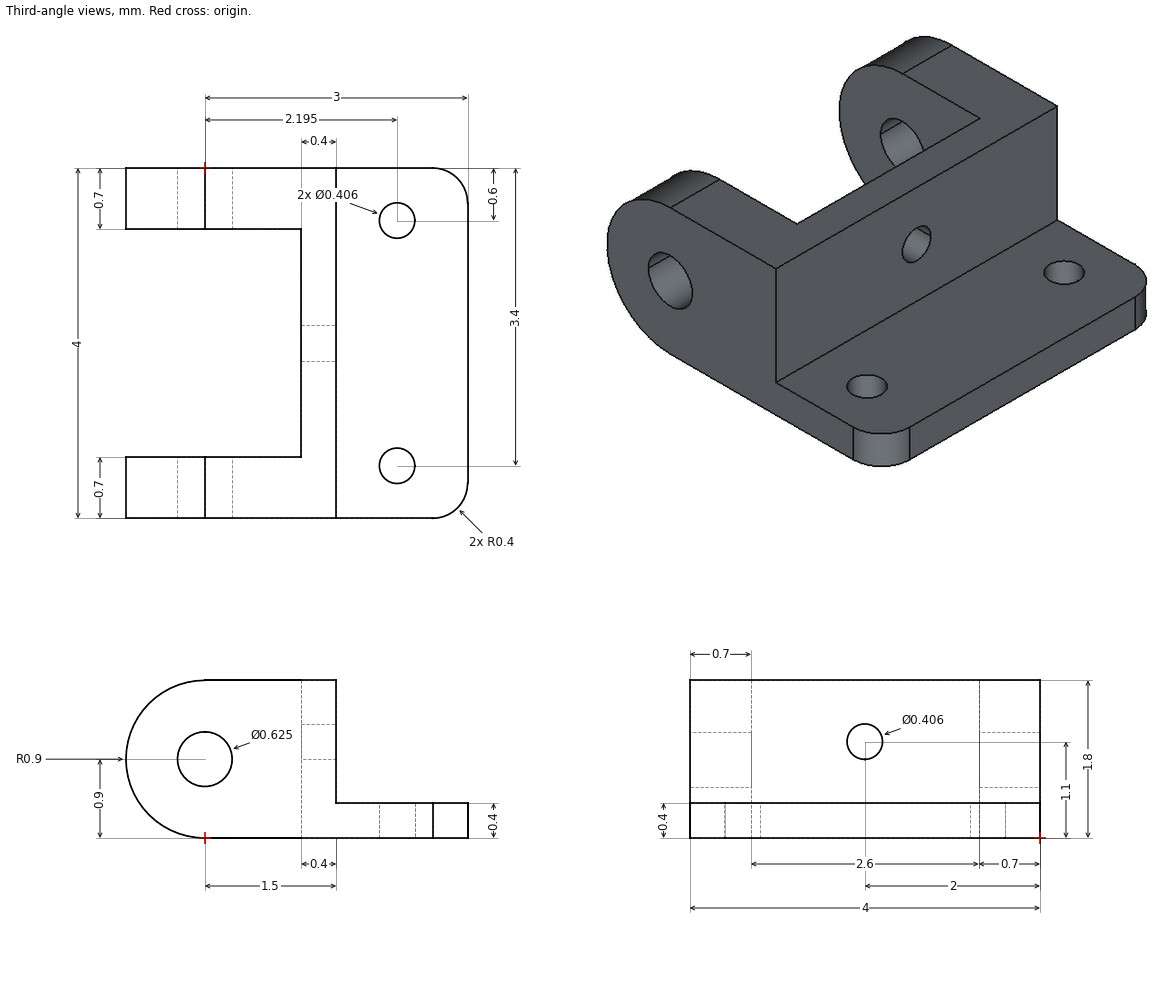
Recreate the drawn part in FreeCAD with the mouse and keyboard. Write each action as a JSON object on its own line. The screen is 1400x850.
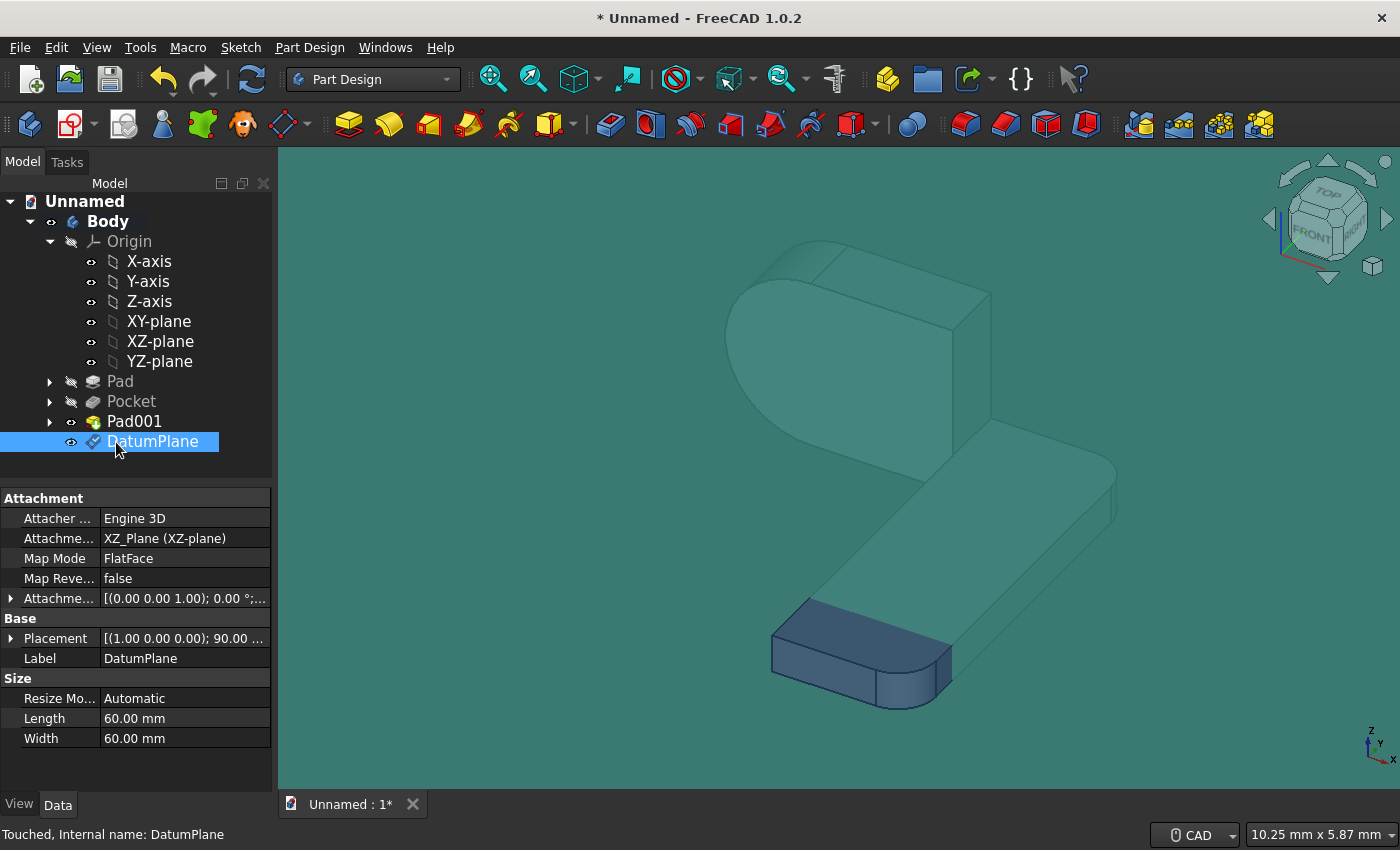
{"action": "left_click", "coordinate": [70, 124]}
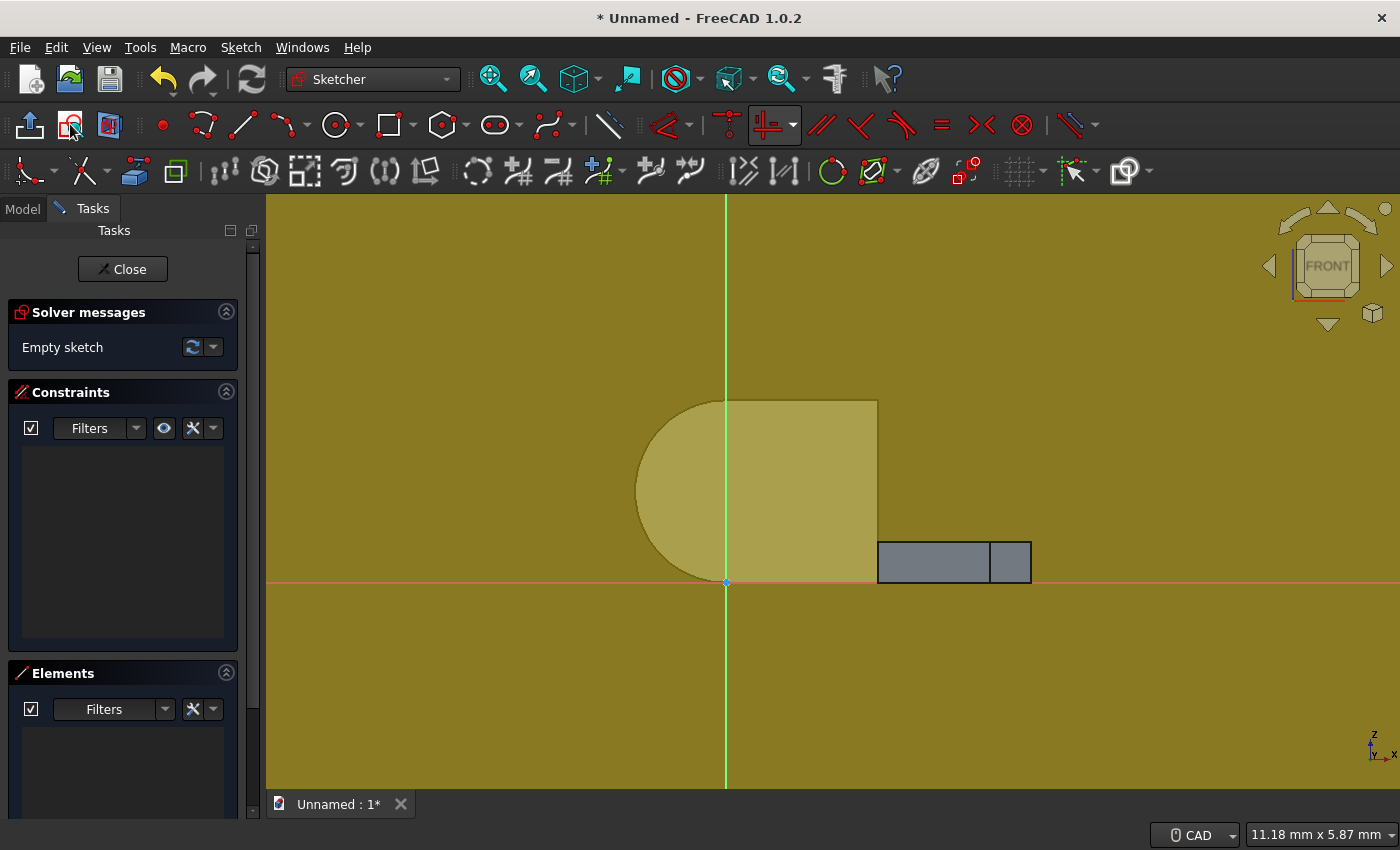
{"action": "key", "text": "q s"}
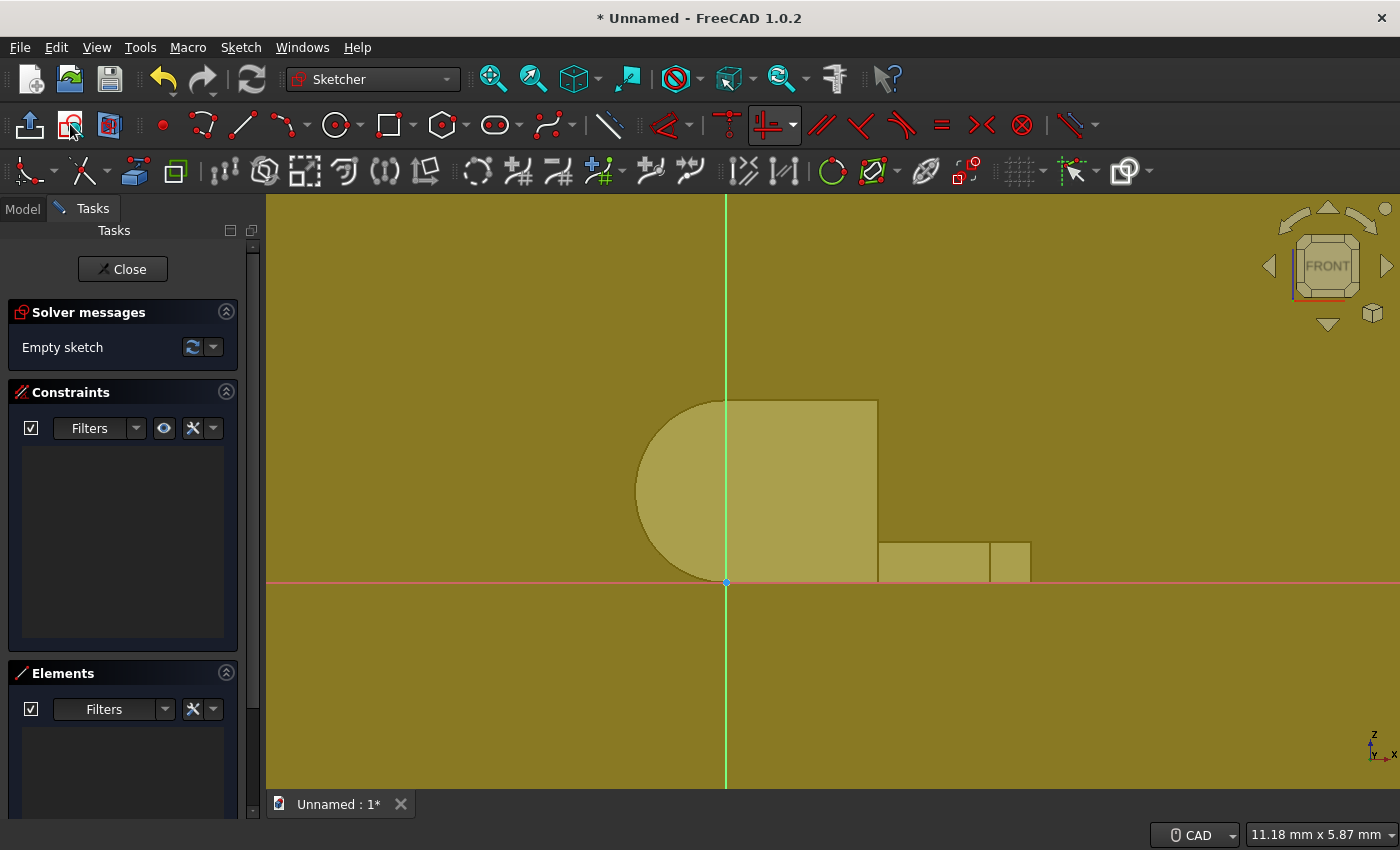
{"action": "scroll", "coordinate": [750, 491], "scroll_direction": "up", "scroll_amount": 4}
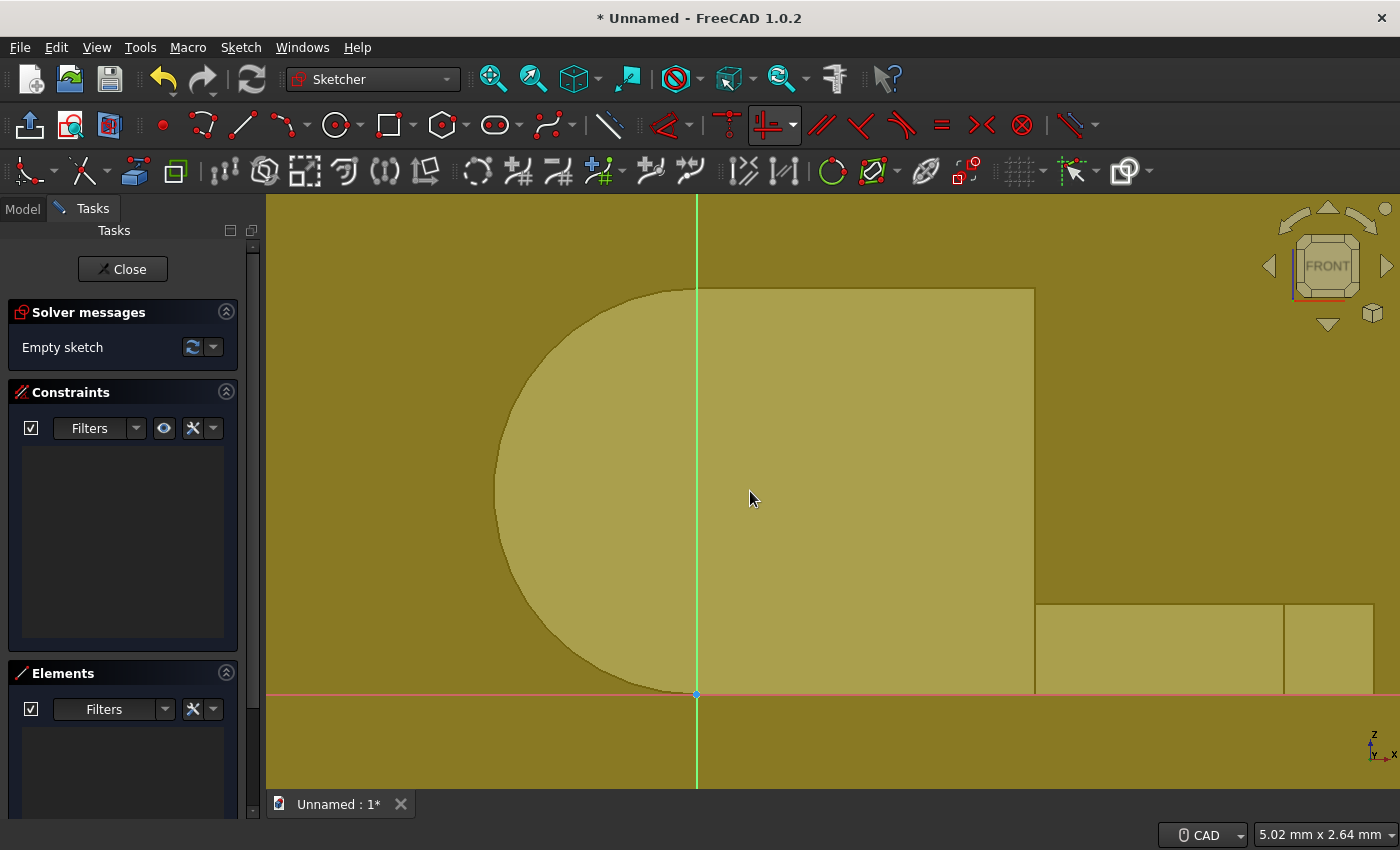
{"action": "key", "text": "g m"}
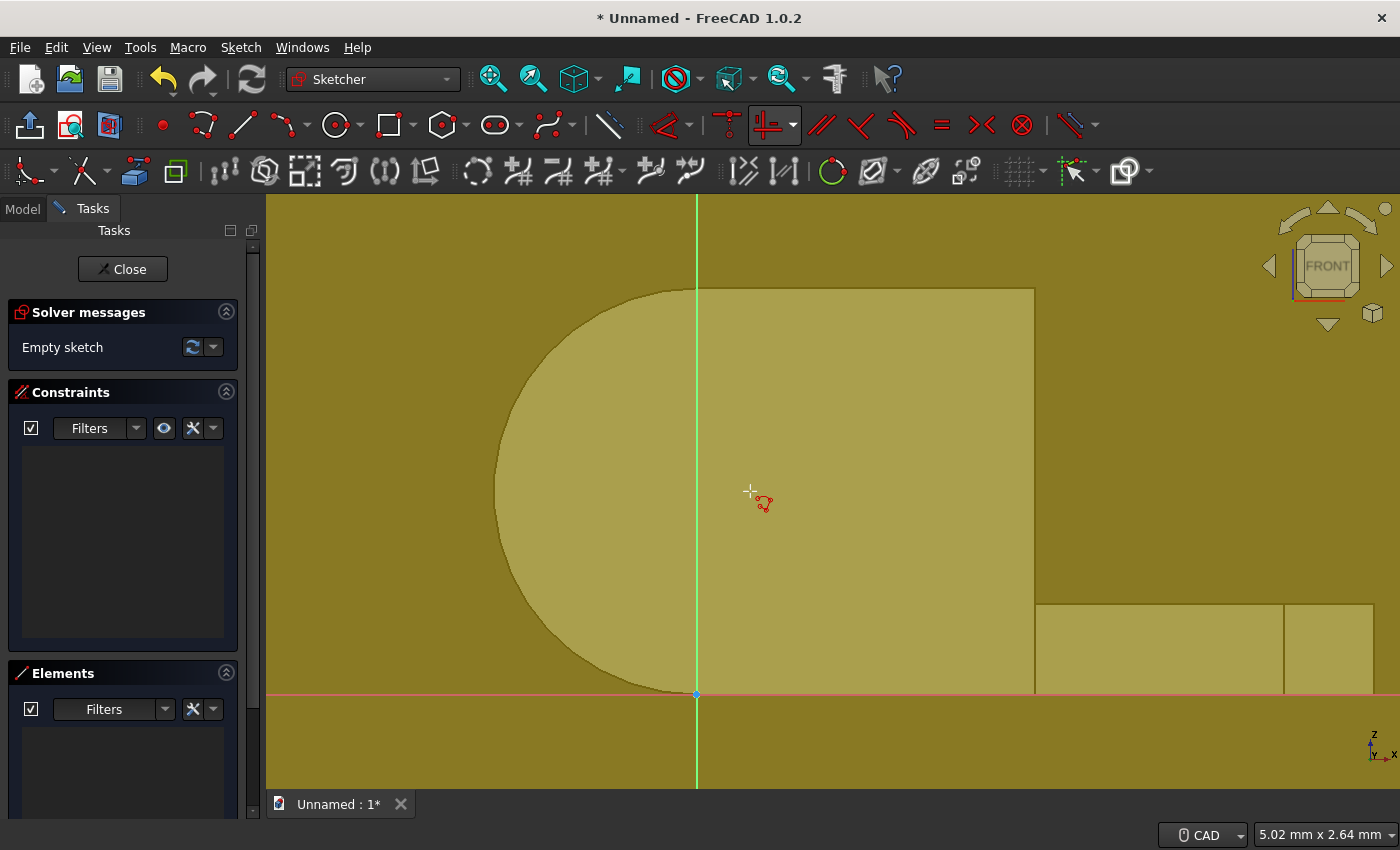
{"action": "left_click", "coordinate": [697, 695]}
{"action": "left_click", "coordinate": [1035, 686]}
{"action": "left_click", "coordinate": [1035, 288]}
{"action": "left_click", "coordinate": [697, 288]}
{"action": "right_click", "coordinate": [697, 288]}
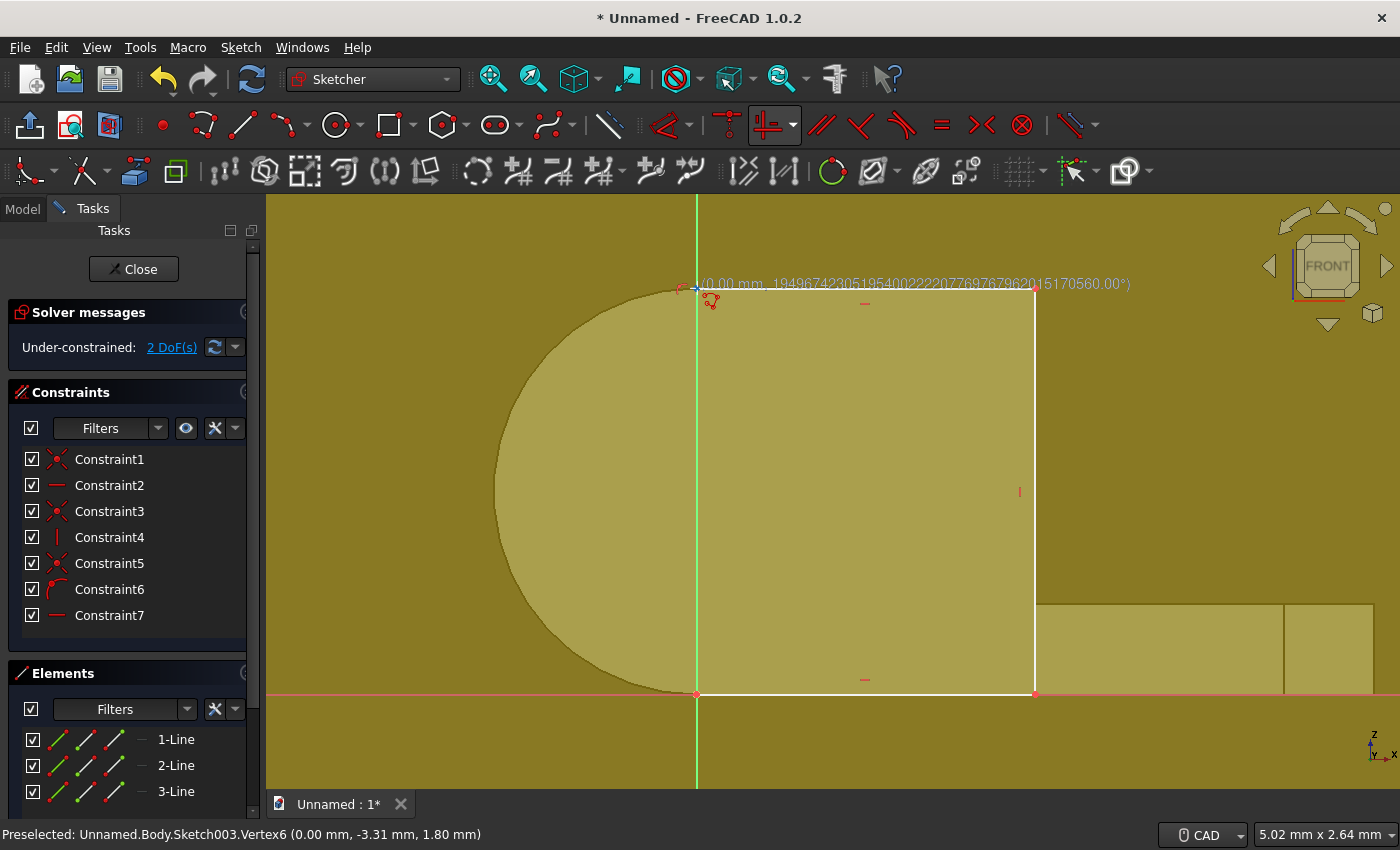
{"action": "left_click", "coordinate": [284, 126]}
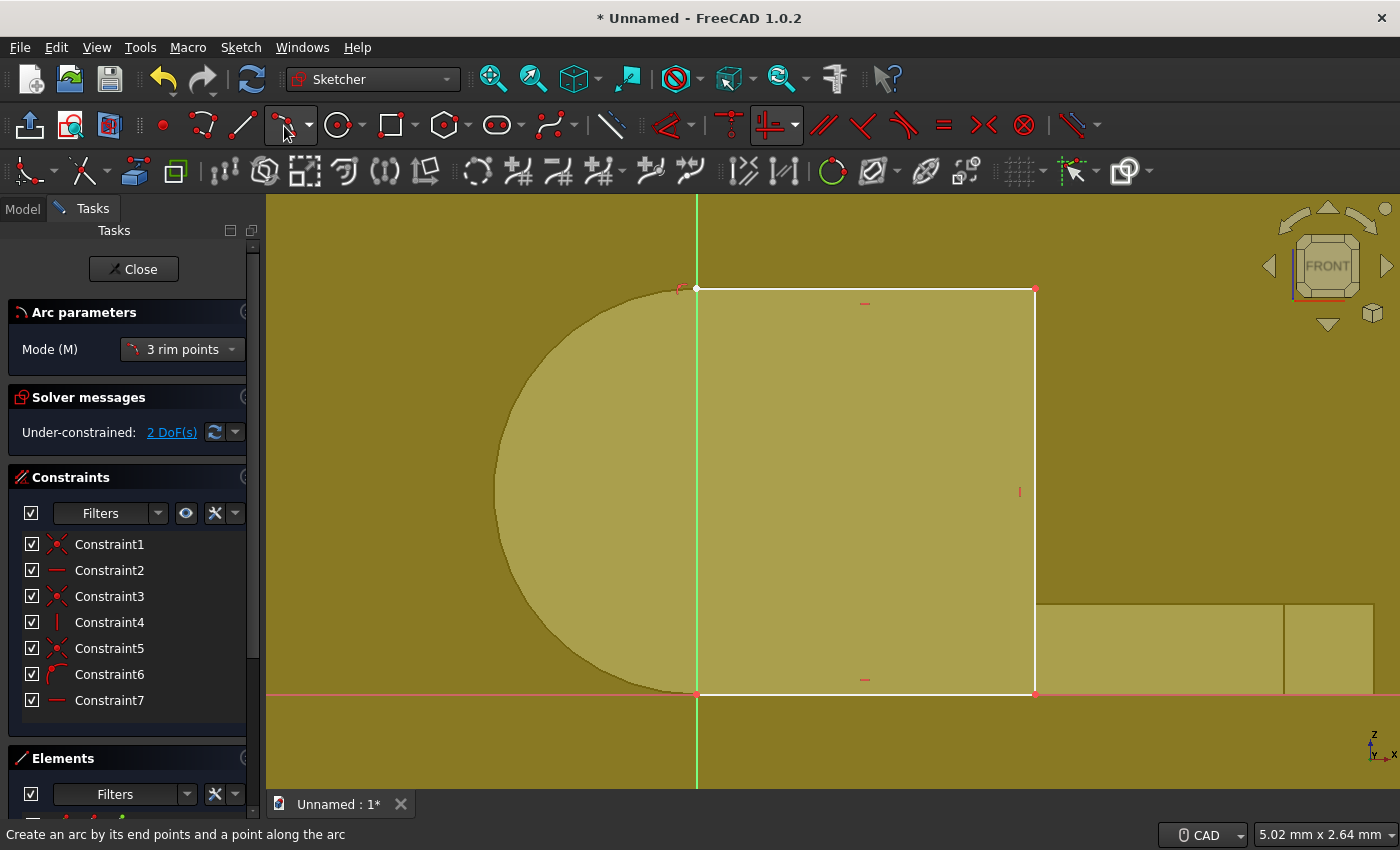
{"action": "left_click", "coordinate": [697, 289]}
{"action": "left_click", "coordinate": [697, 695]}
{"action": "left_click", "coordinate": [494, 491]}
{"action": "key", "text": "Escape"}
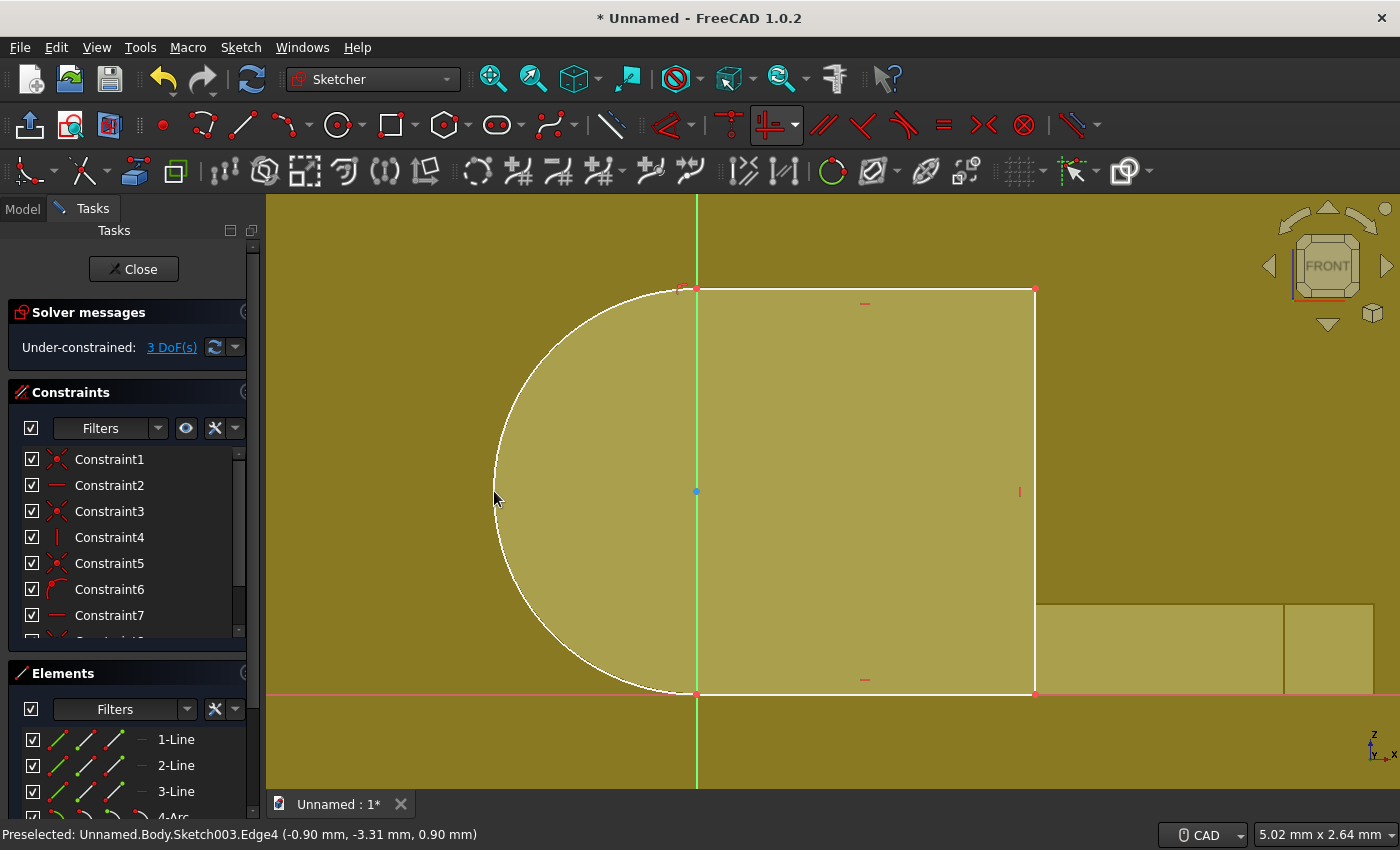
{"action": "left_click", "coordinate": [798, 695]}